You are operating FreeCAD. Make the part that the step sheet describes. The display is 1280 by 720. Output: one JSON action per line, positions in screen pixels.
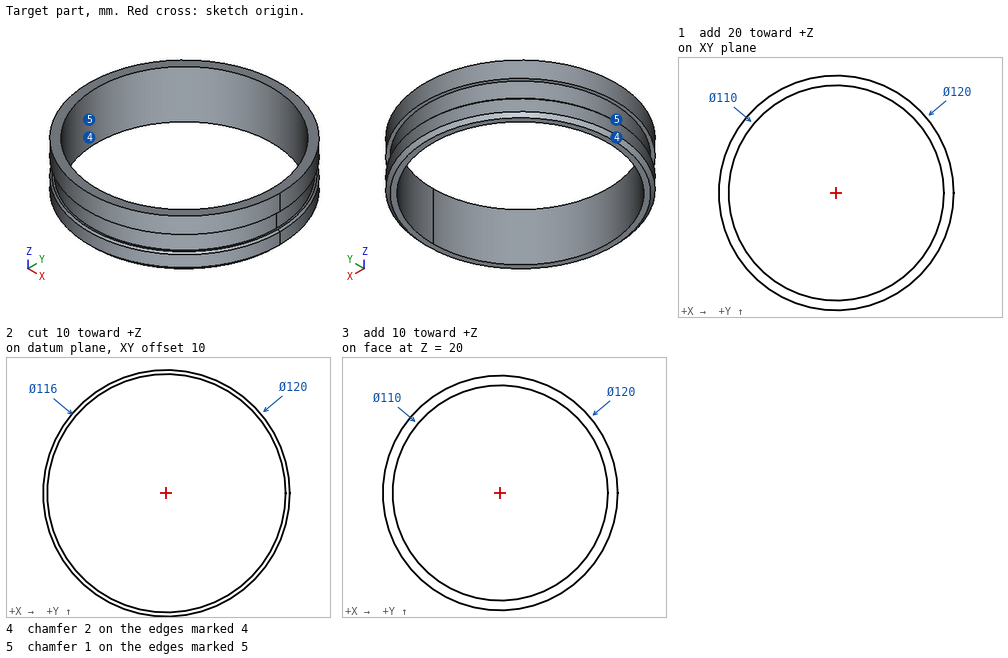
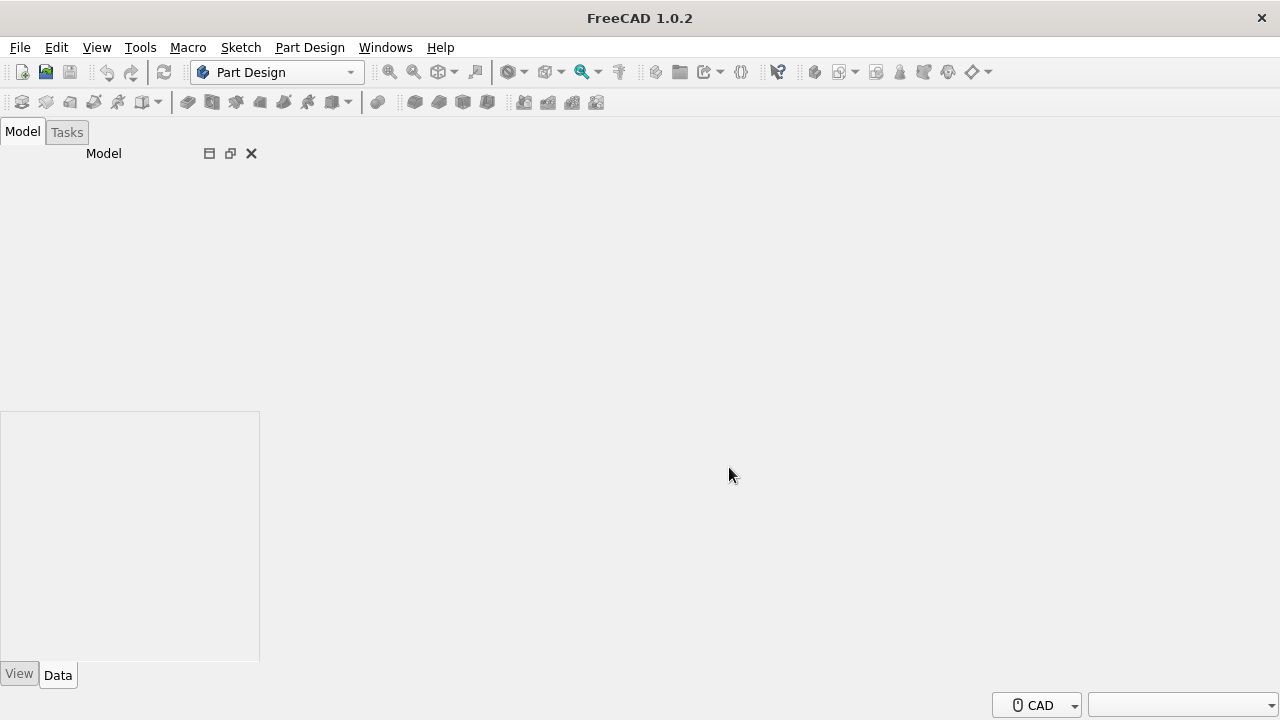
{"action": "key", "text": "ctrl+n"}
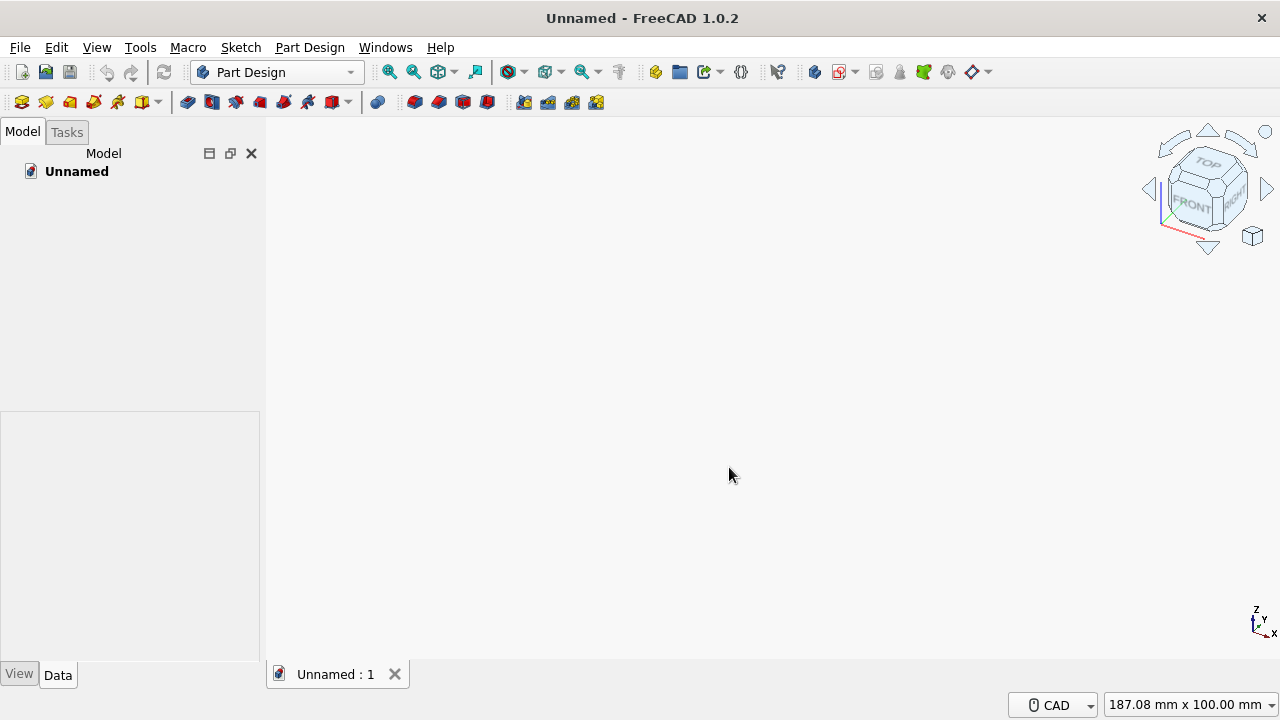
{"action": "left_click", "coordinate": [840, 72]}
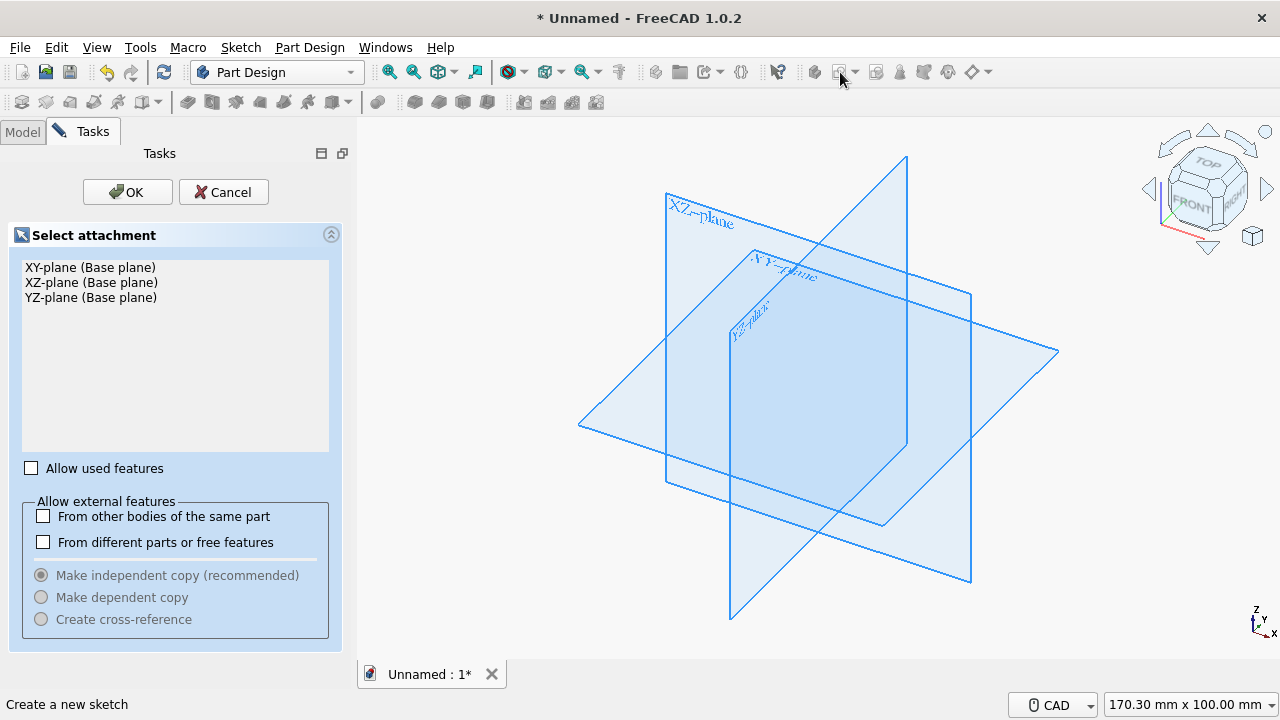
{"action": "left_click", "coordinate": [82, 268]}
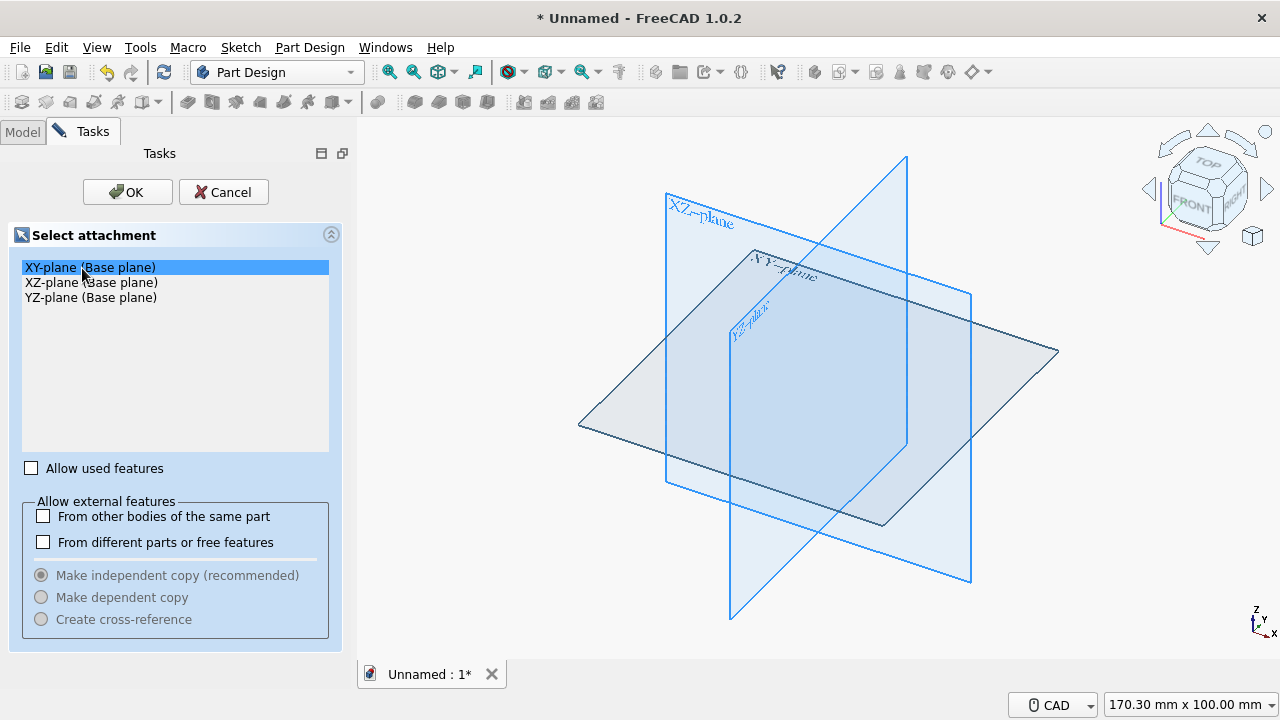
{"action": "left_click", "coordinate": [128, 192]}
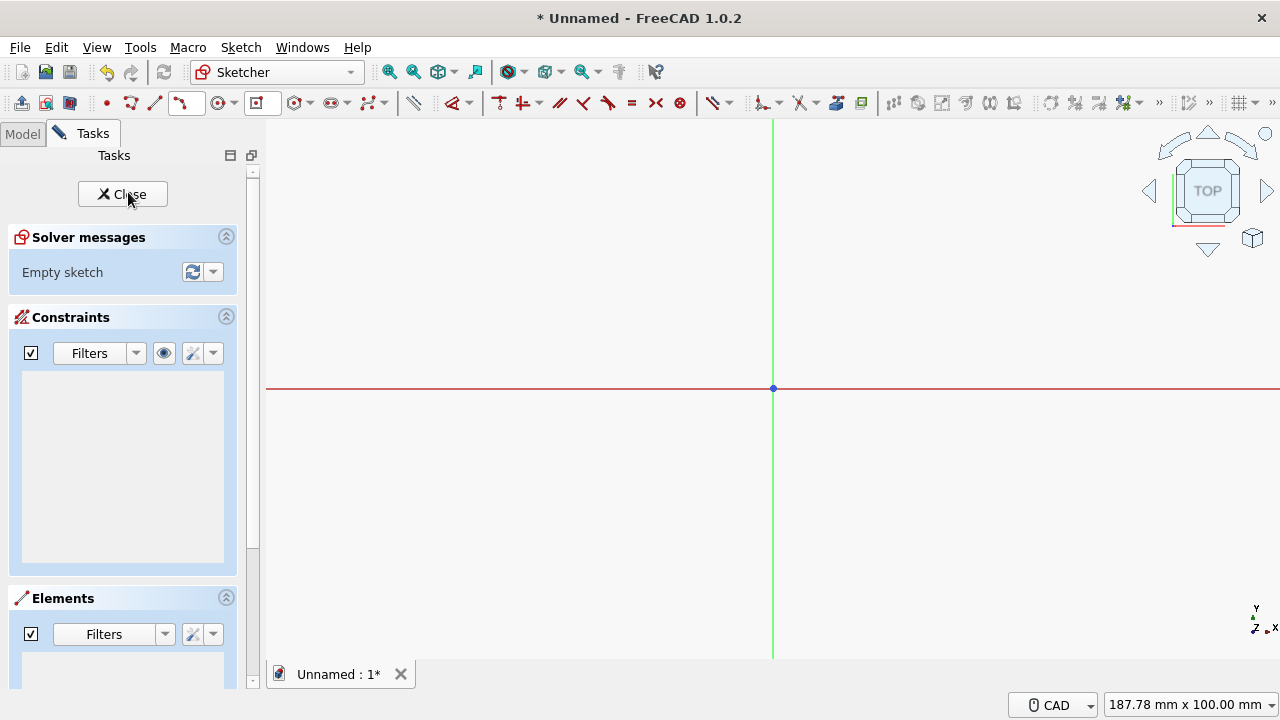
{"action": "scroll", "coordinate": [621, 389], "scroll_direction": "down", "scroll_amount": 3}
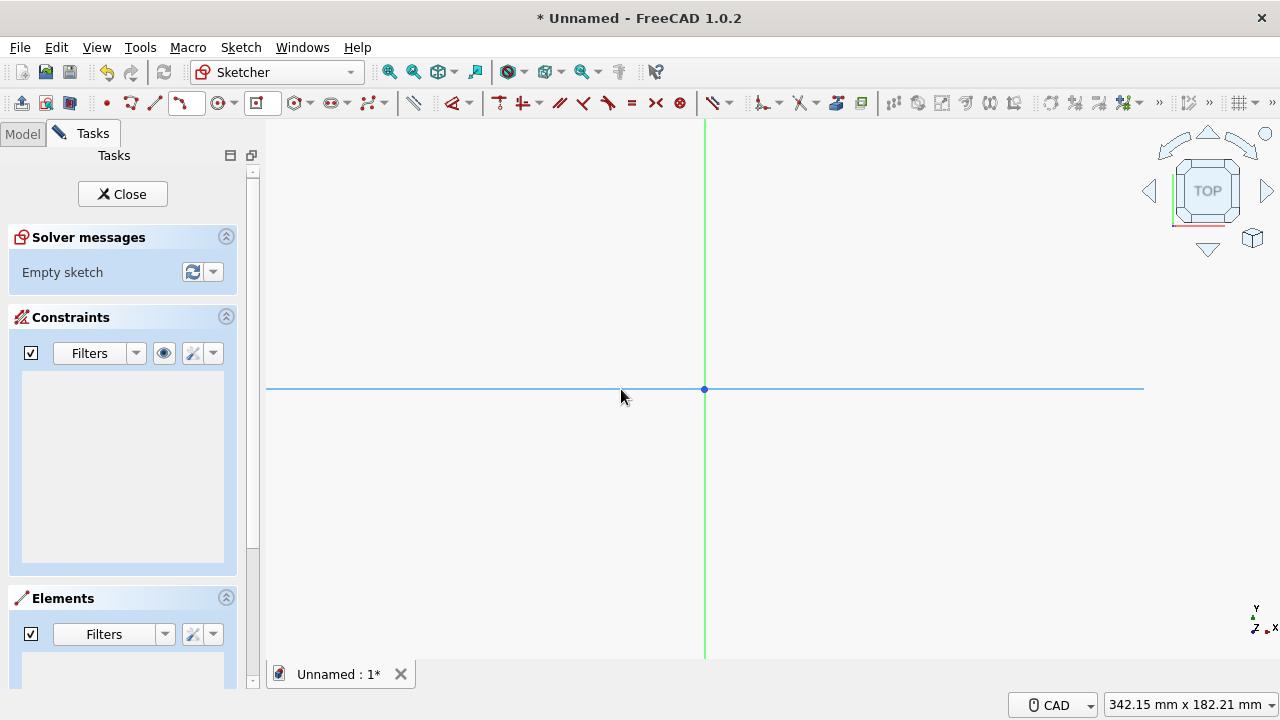
{"action": "key", "text": "g c"}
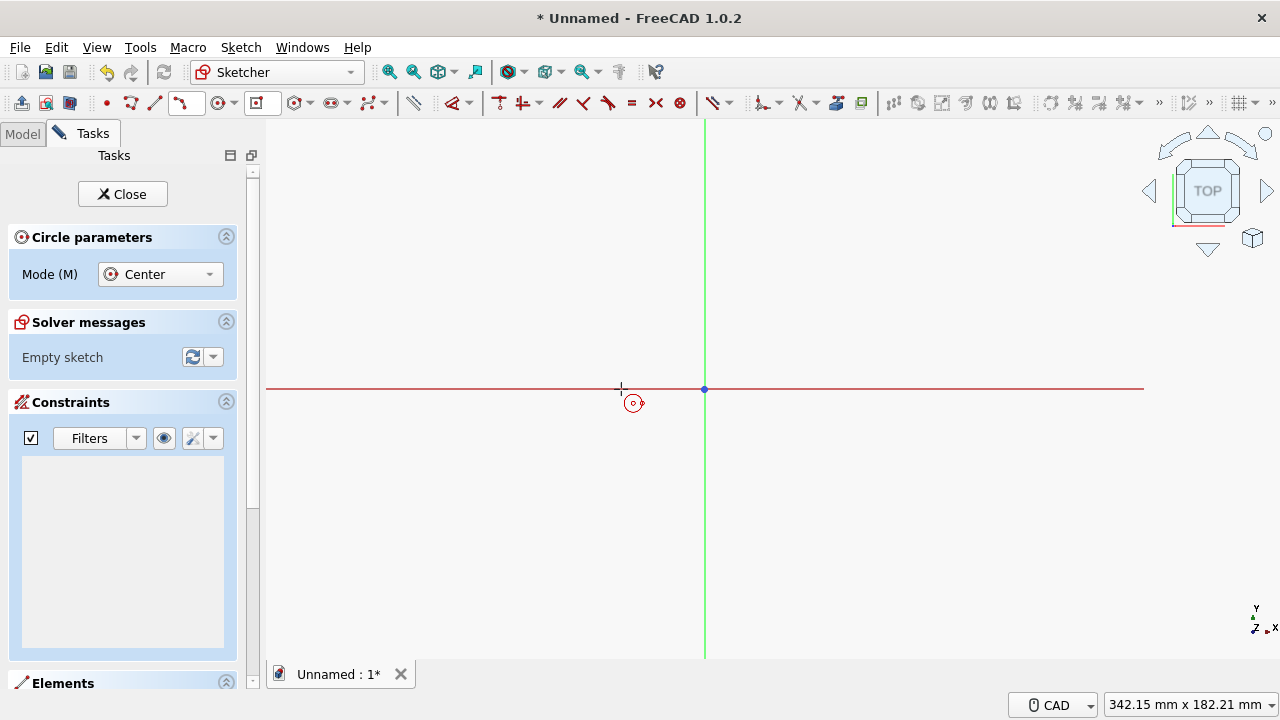
{"action": "left_click", "coordinate": [705, 389]}
{"action": "left_click", "coordinate": [830, 263]}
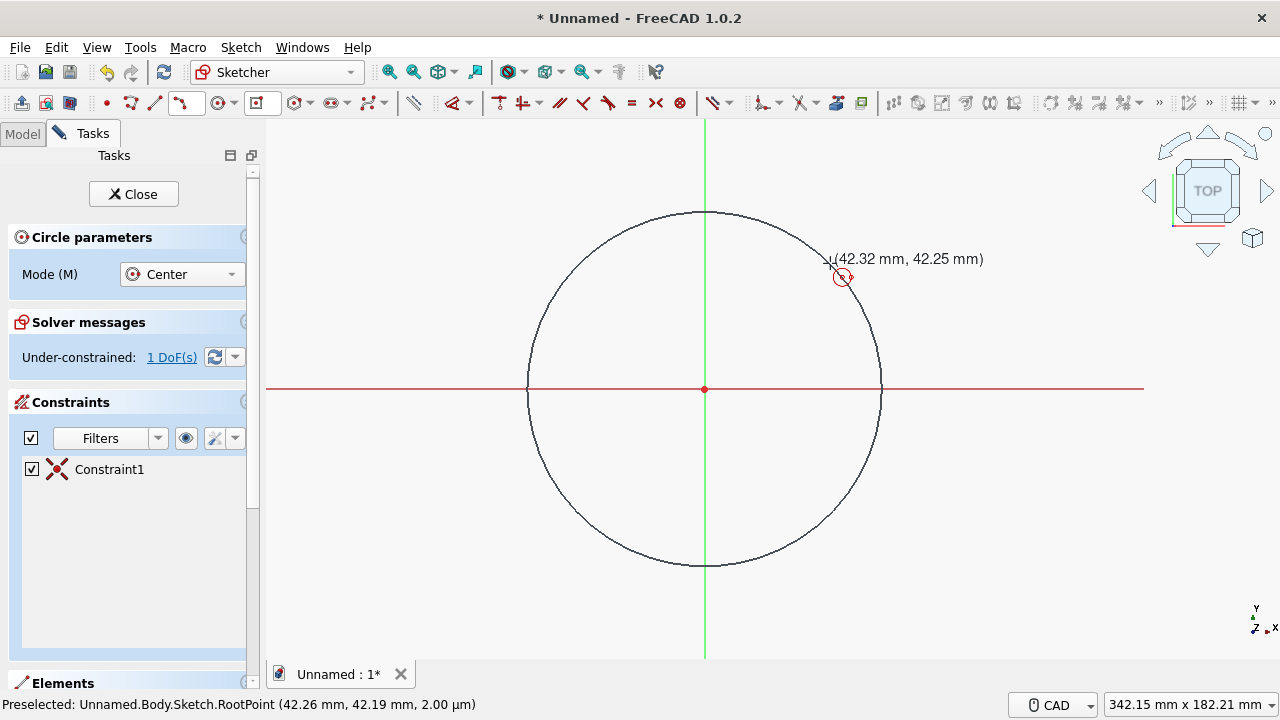
{"action": "left_click", "coordinate": [705, 389]}
{"action": "left_click", "coordinate": [820, 274]}
{"action": "key", "text": "Escape"}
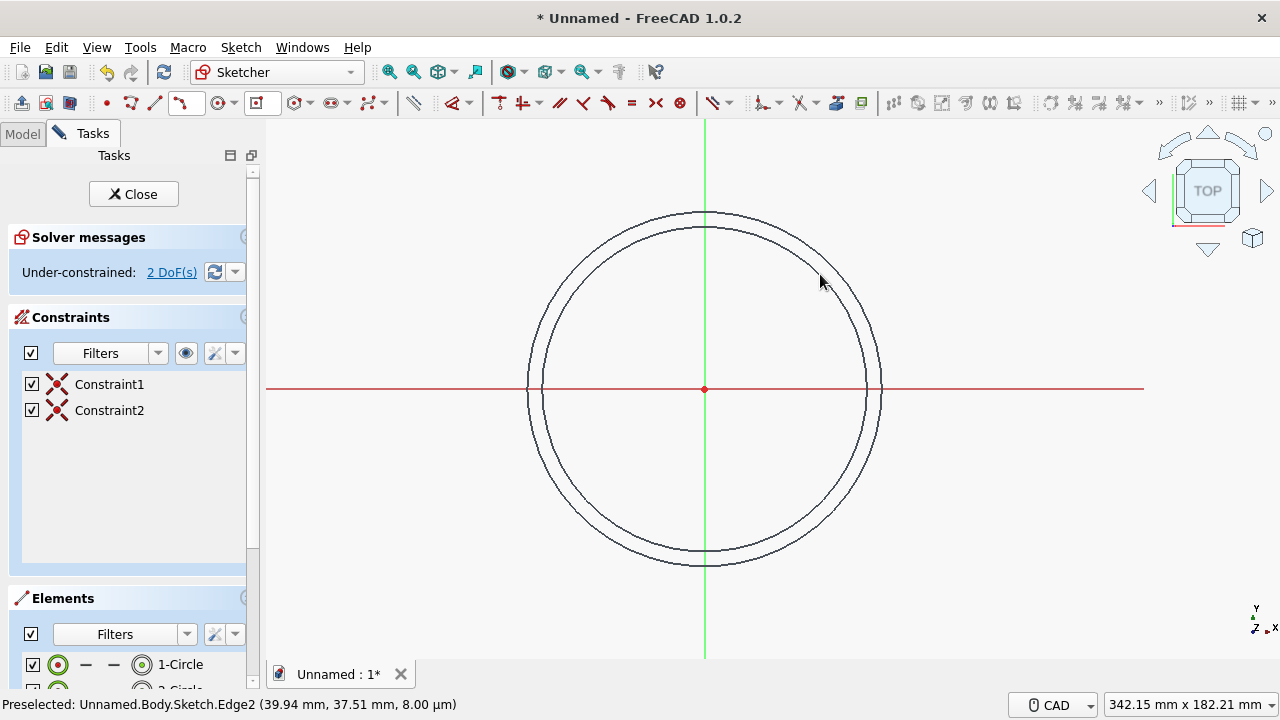
{"action": "left_click", "coordinate": [830, 264]}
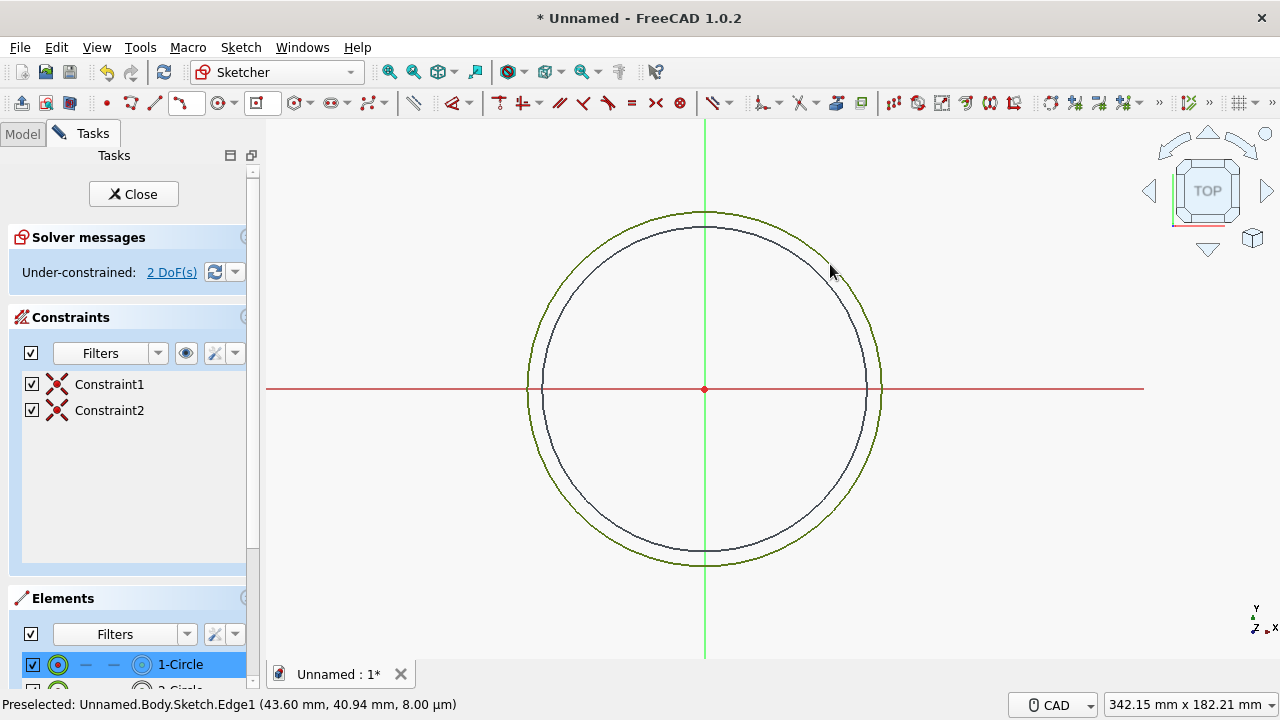
{"action": "key", "text": "k o"}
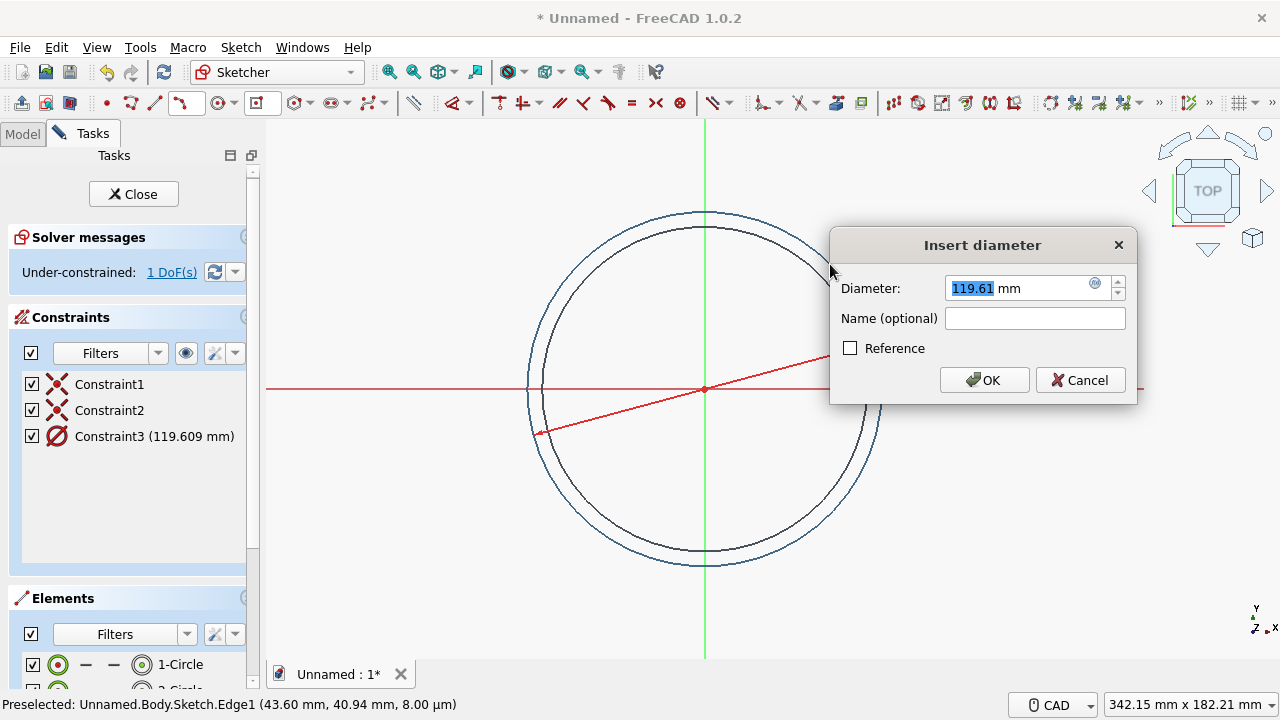
{"action": "type", "text": "120"}
{"action": "key", "text": "Return"}